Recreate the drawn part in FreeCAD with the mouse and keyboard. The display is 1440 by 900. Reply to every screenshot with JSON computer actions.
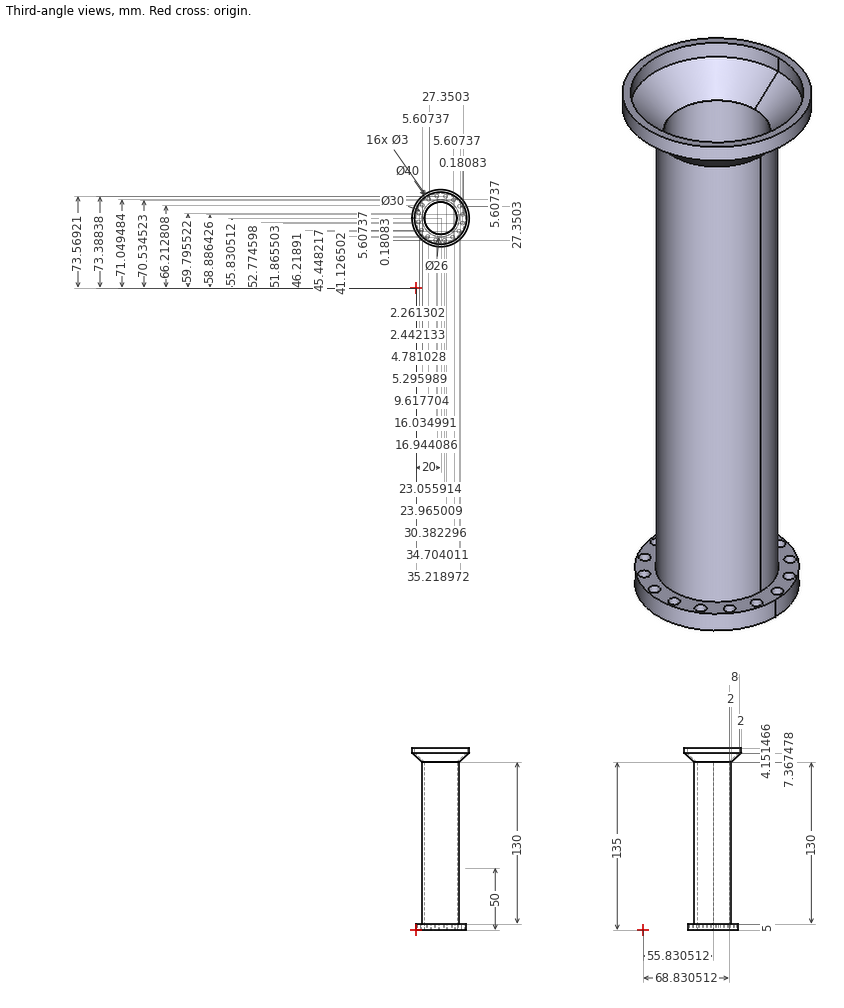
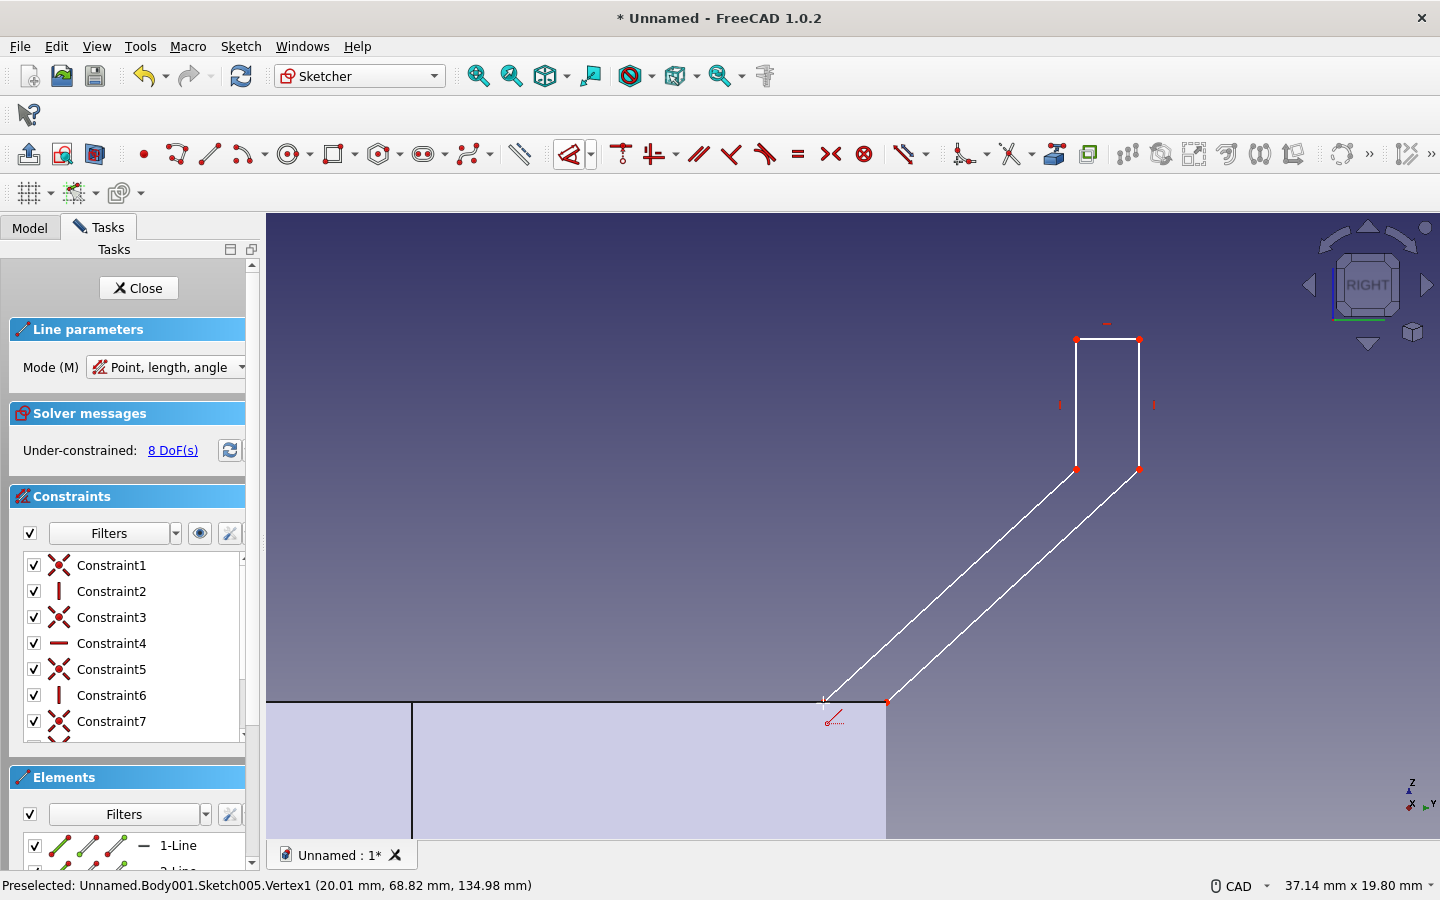
{"action": "left_click", "coordinate": [412, 739]}
{"action": "left_click", "coordinate": [412, 302]}
{"action": "key", "text": "Escape"}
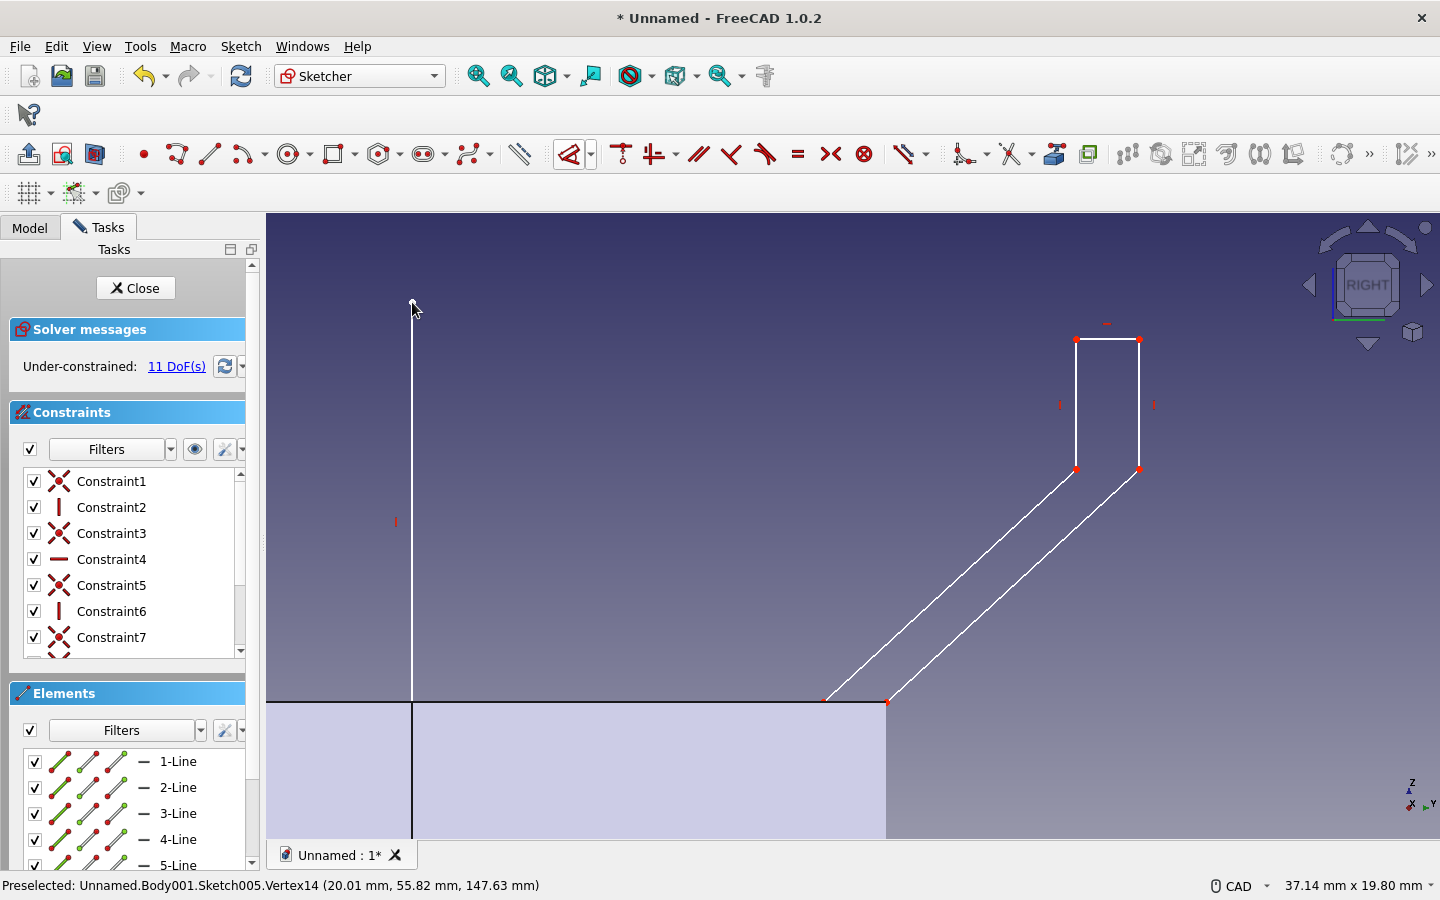
{"action": "left_click", "coordinate": [412, 609]}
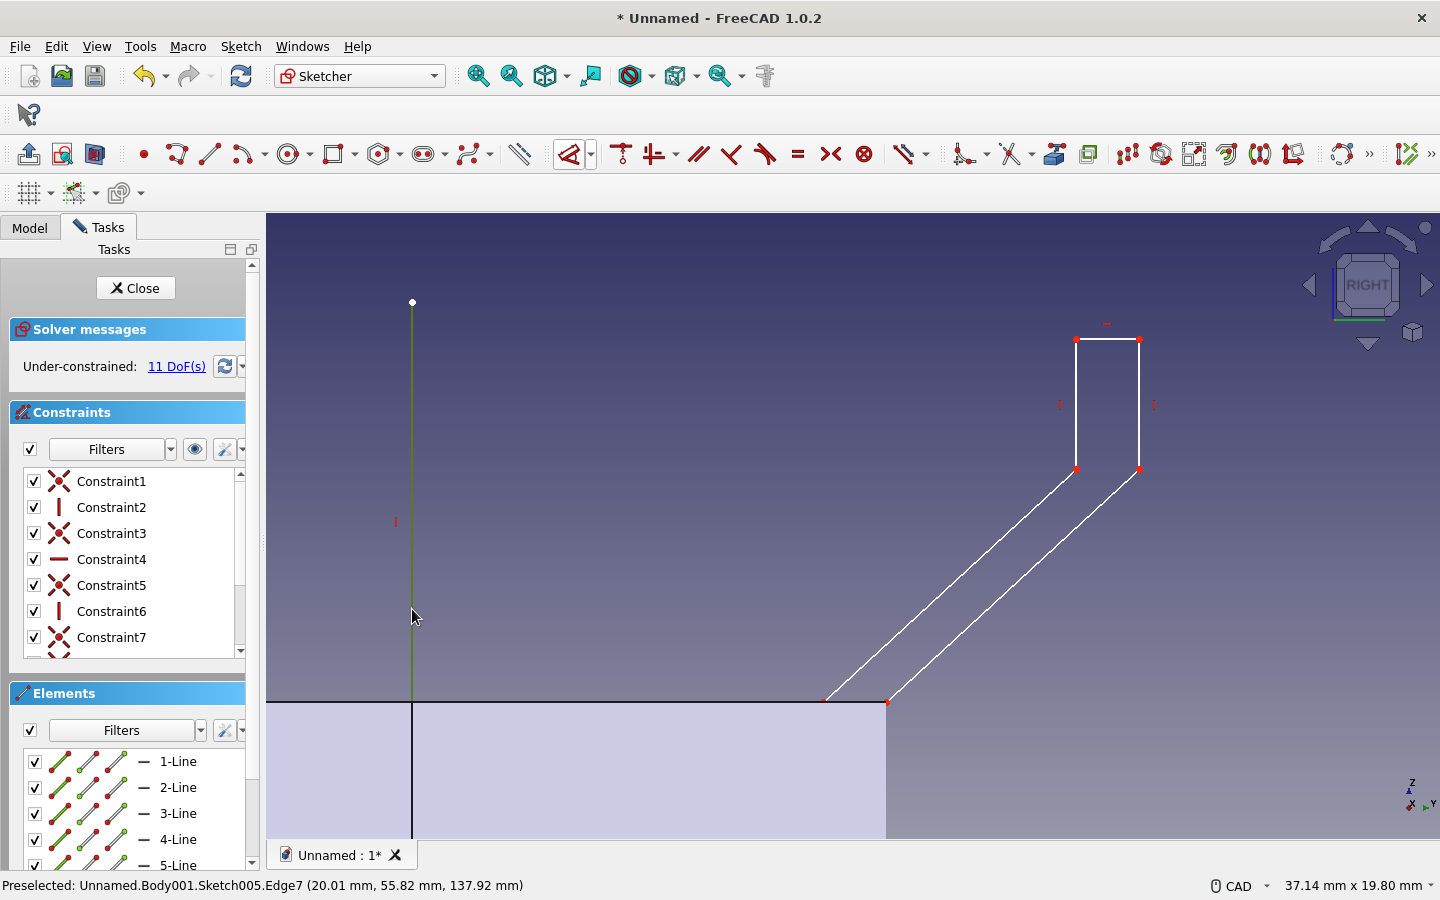
{"action": "left_click", "coordinate": [520, 154]}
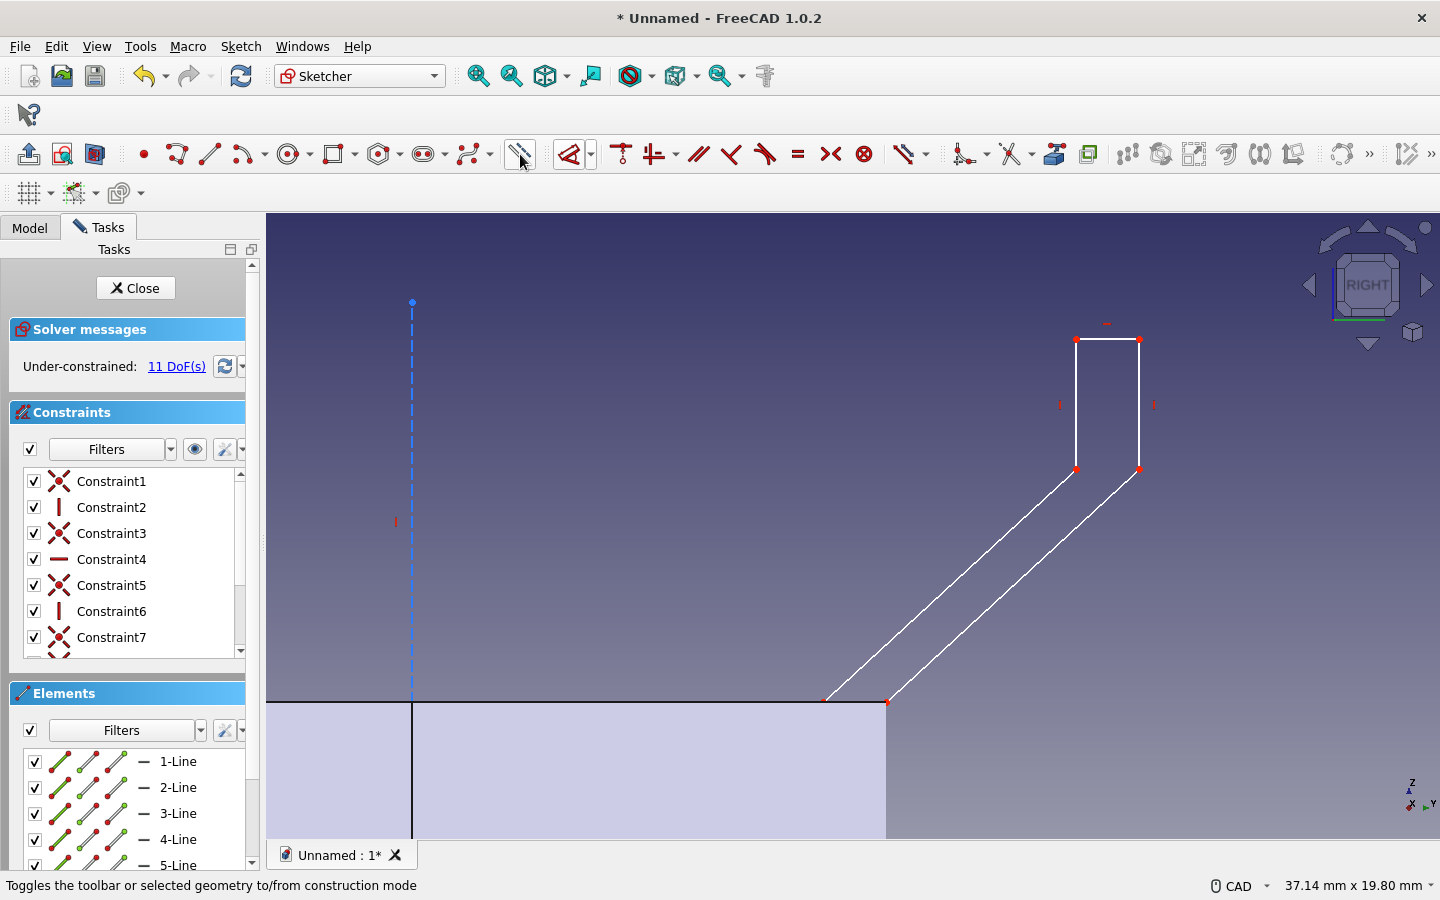
{"action": "left_click", "coordinate": [1095, 339]}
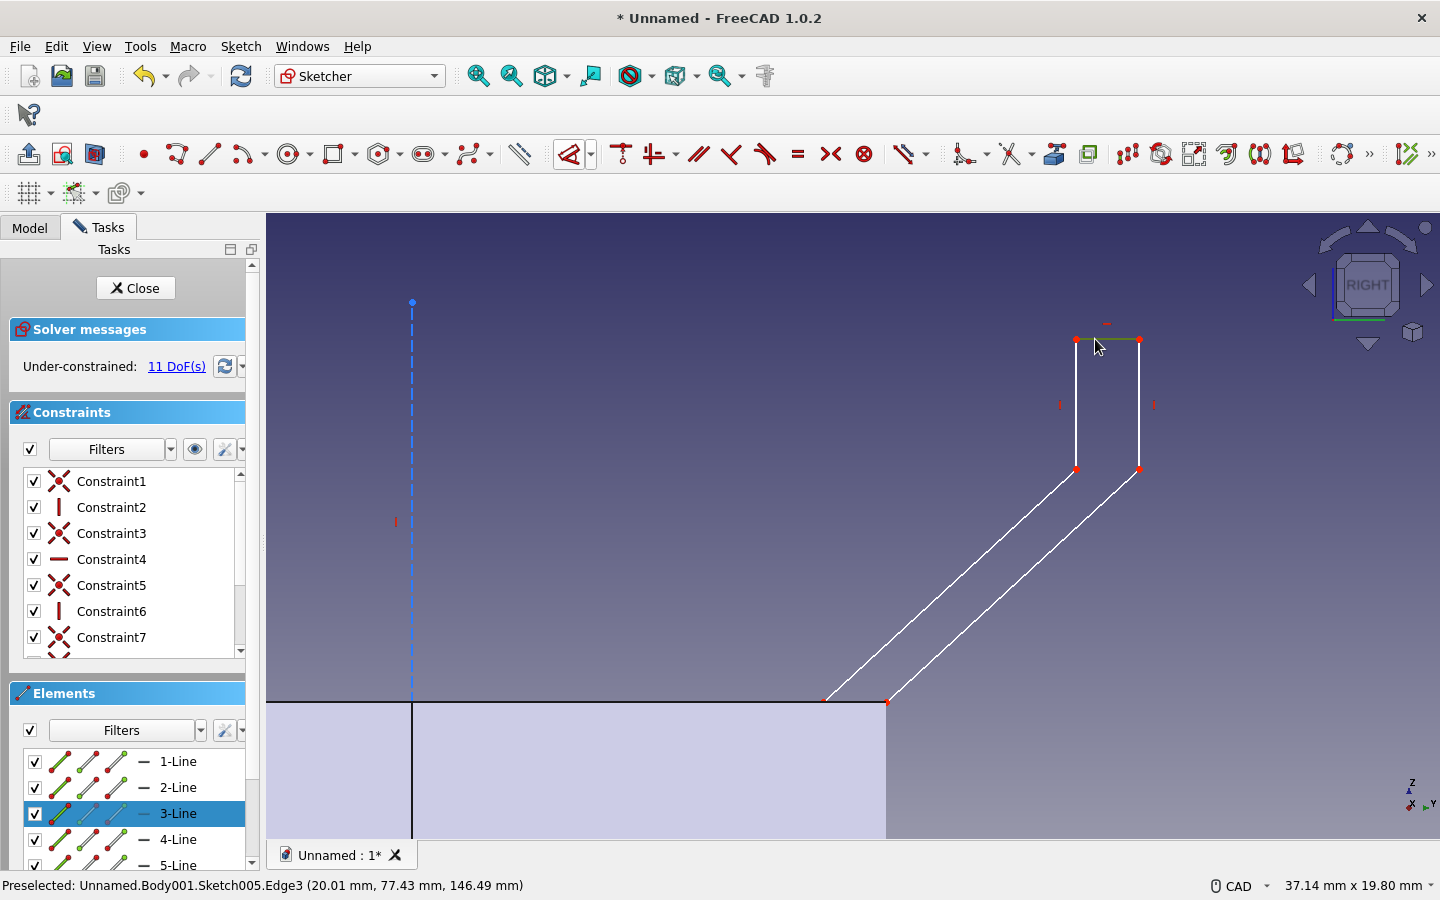
{"action": "key", "text": "l"}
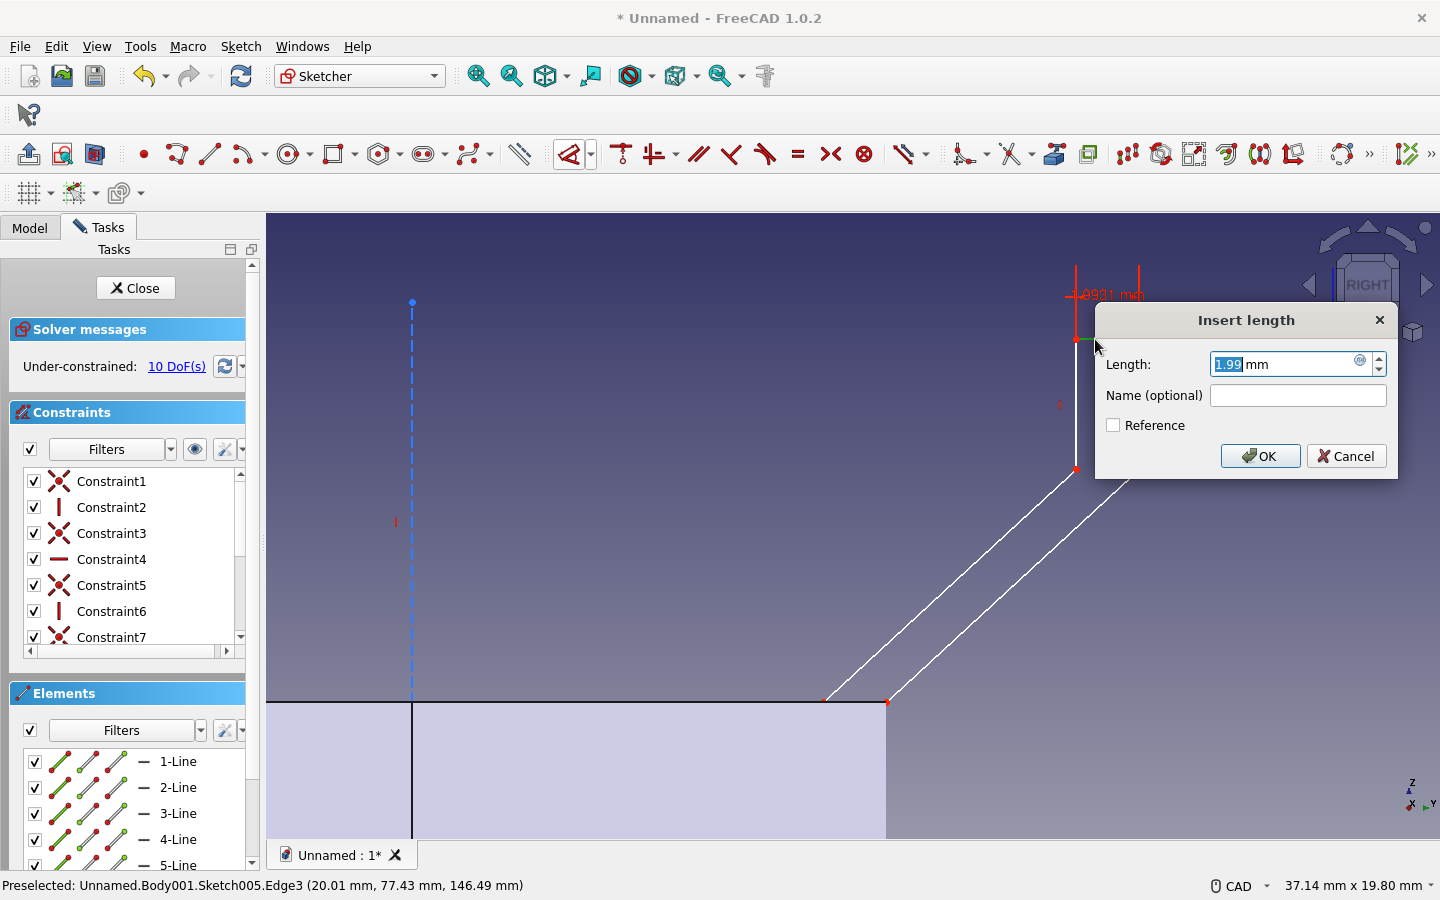
{"action": "type", "text": "2"}
{"action": "key", "text": "Return"}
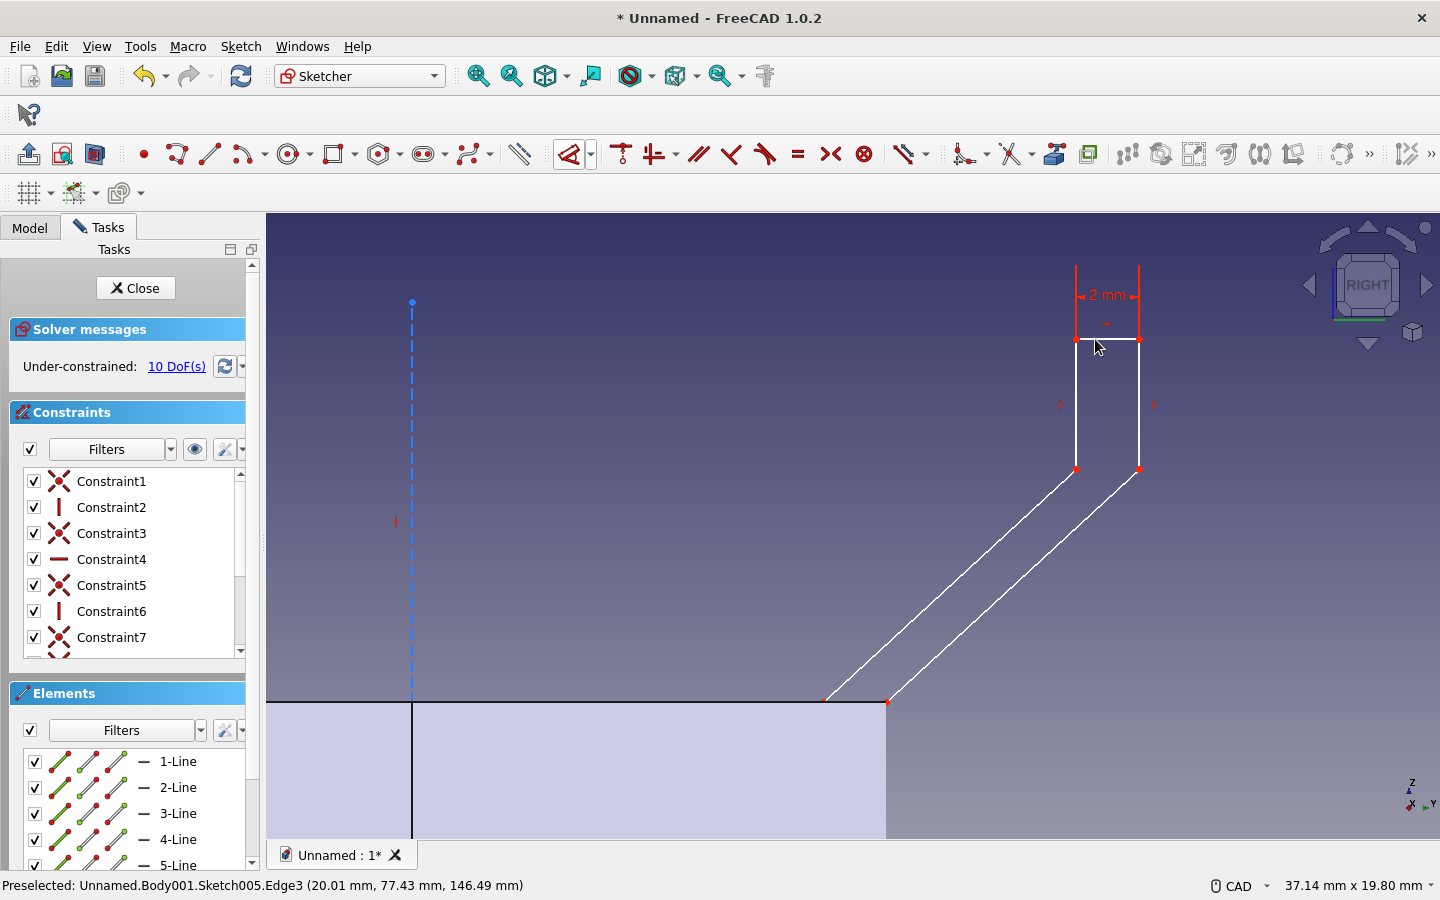
{"action": "left_click", "coordinate": [867, 703]}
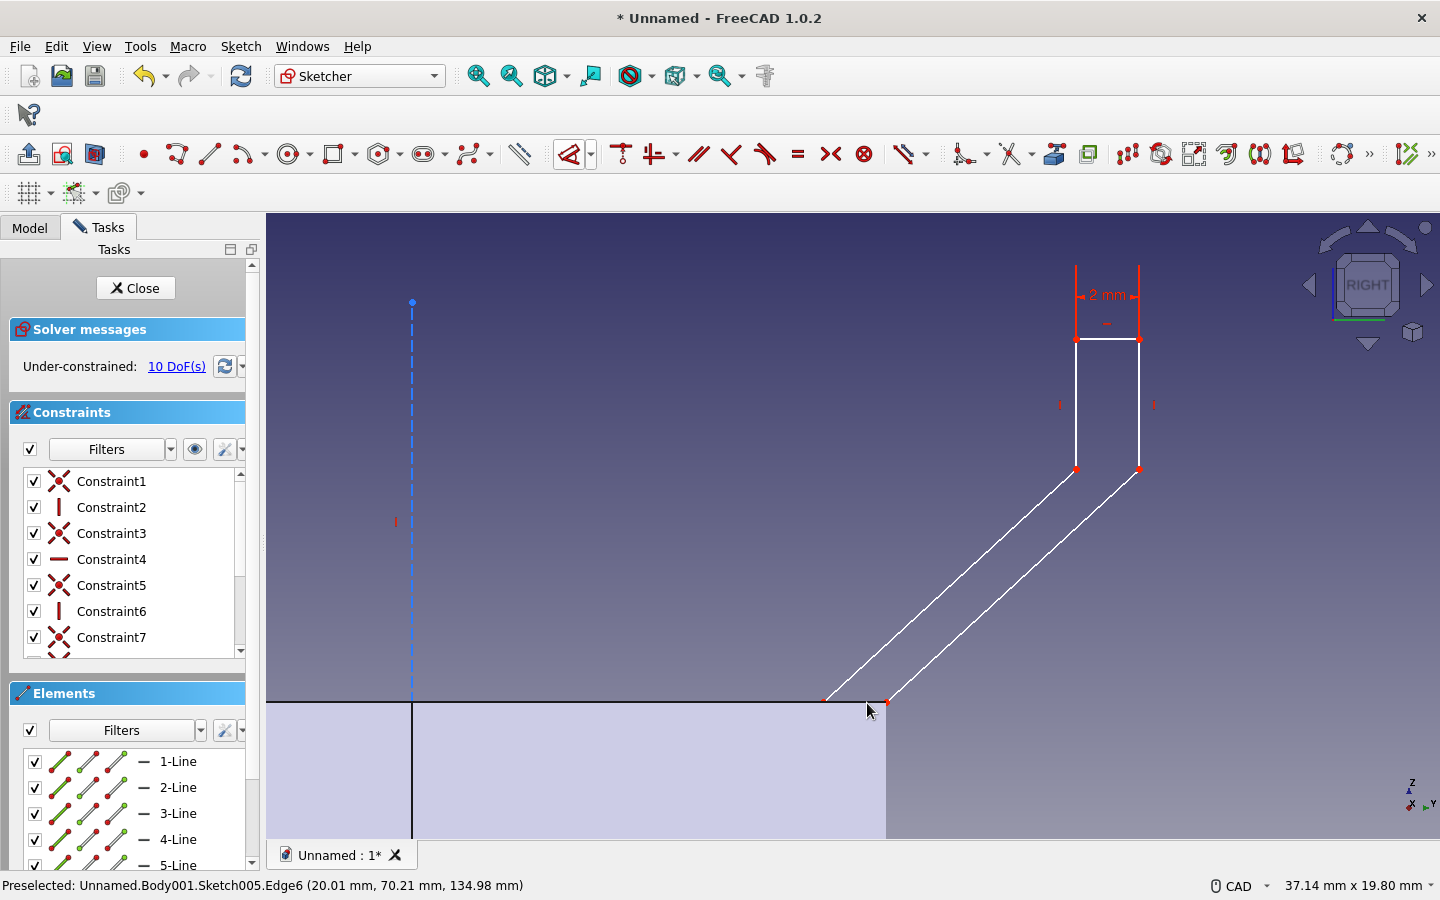
{"action": "left_click", "coordinate": [590, 154]}